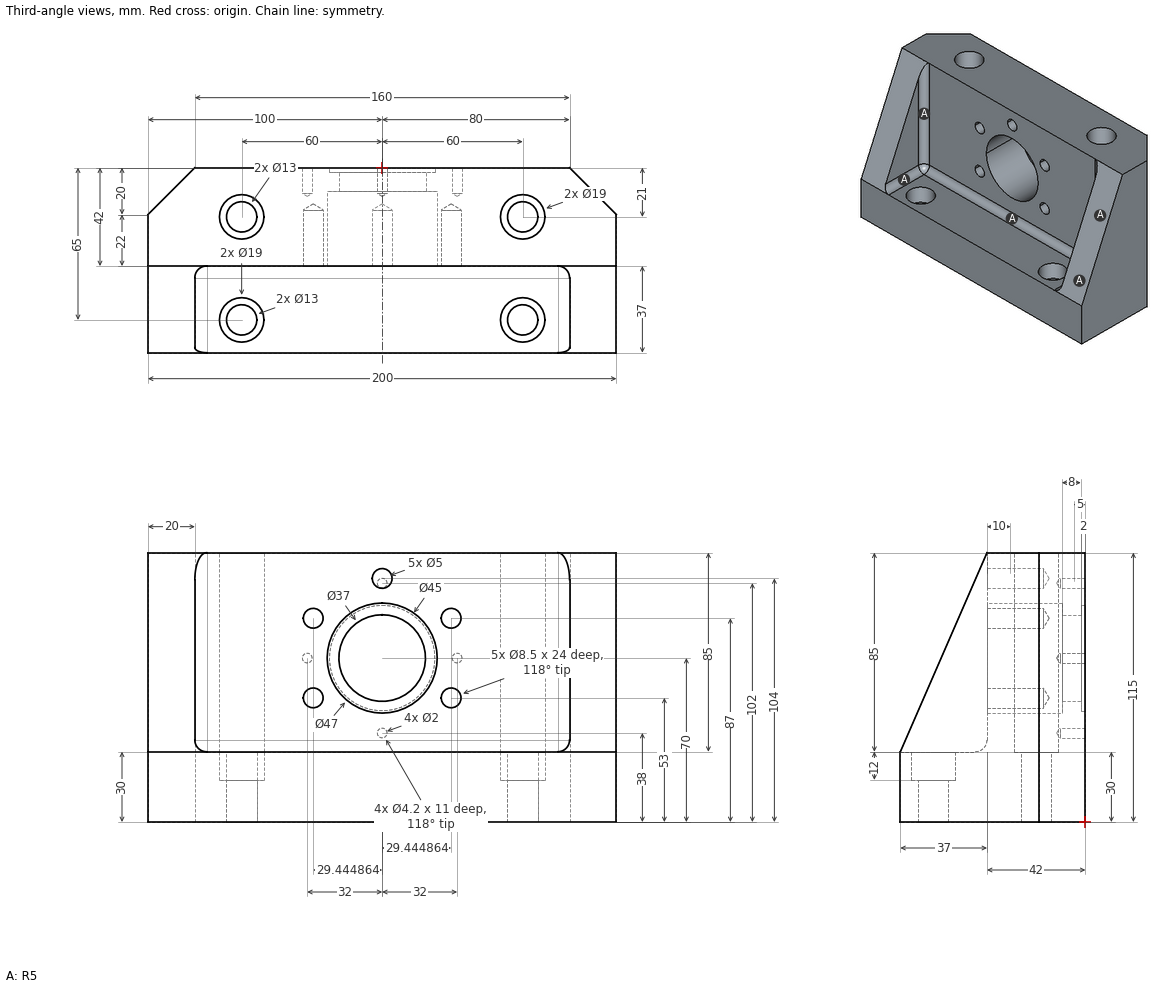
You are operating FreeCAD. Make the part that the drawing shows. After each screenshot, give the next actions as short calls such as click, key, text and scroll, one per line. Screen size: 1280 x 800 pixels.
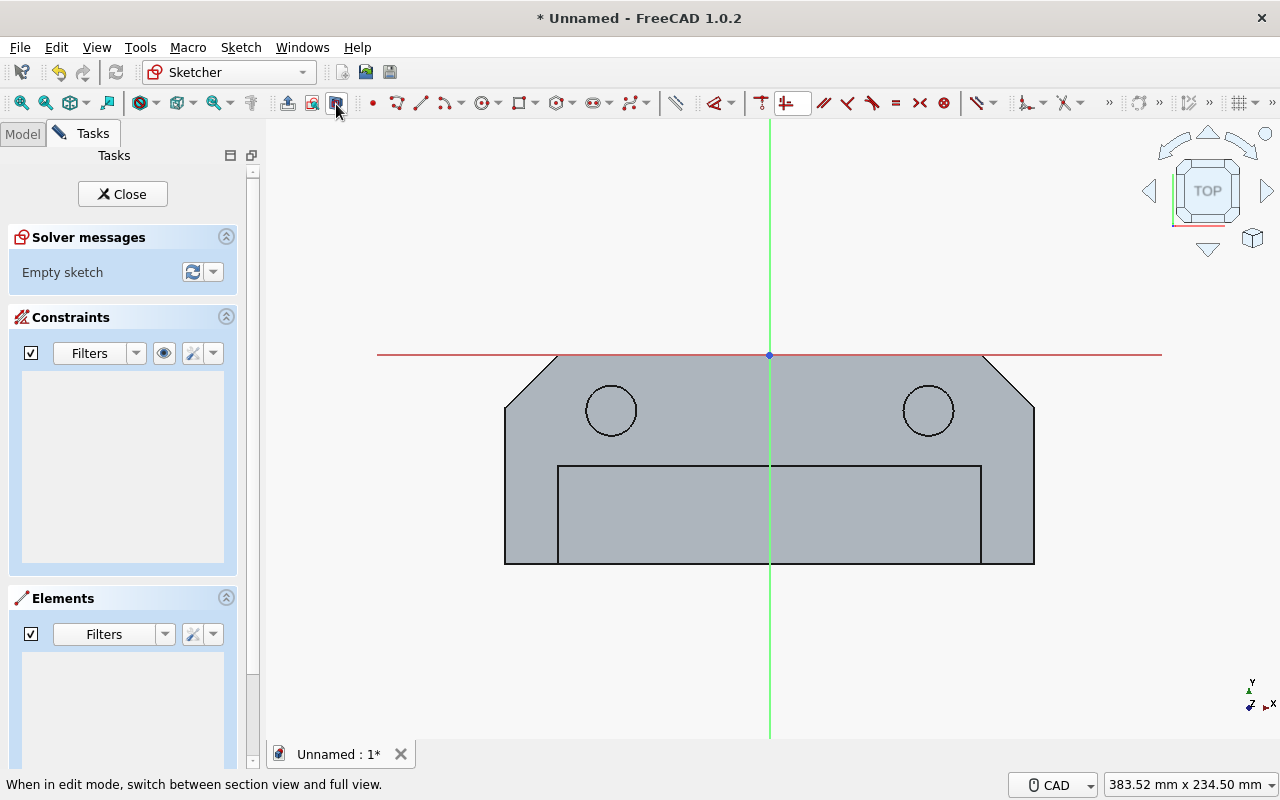
scroll(903, 315, up, 2)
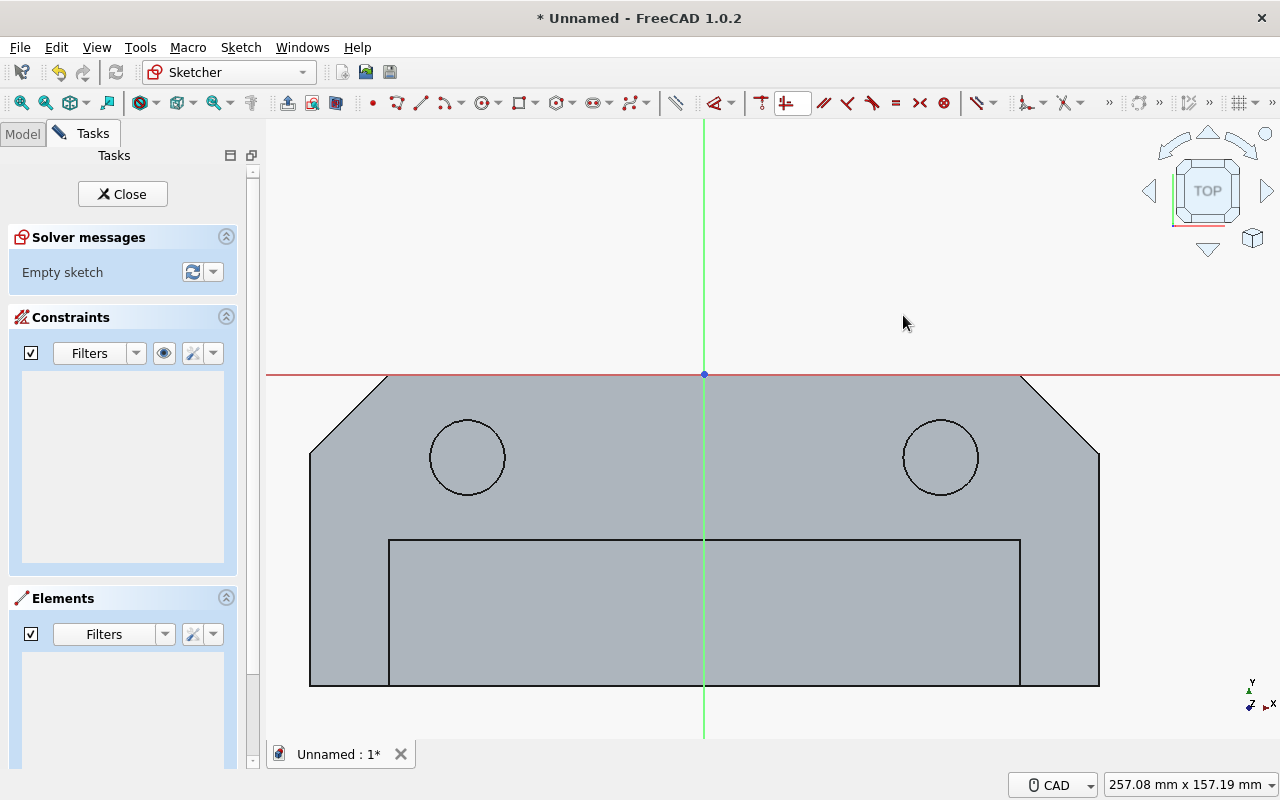
click(482, 104)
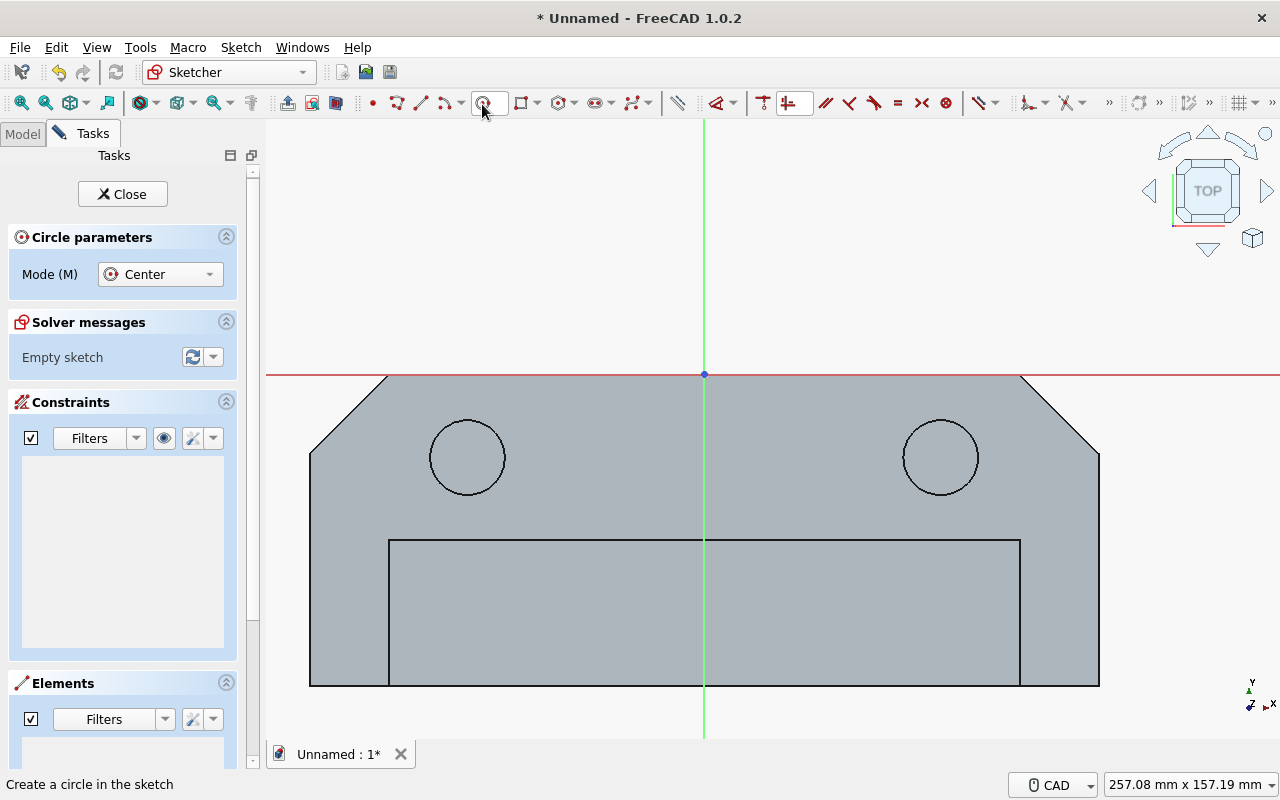
click(467, 458)
move(486, 440)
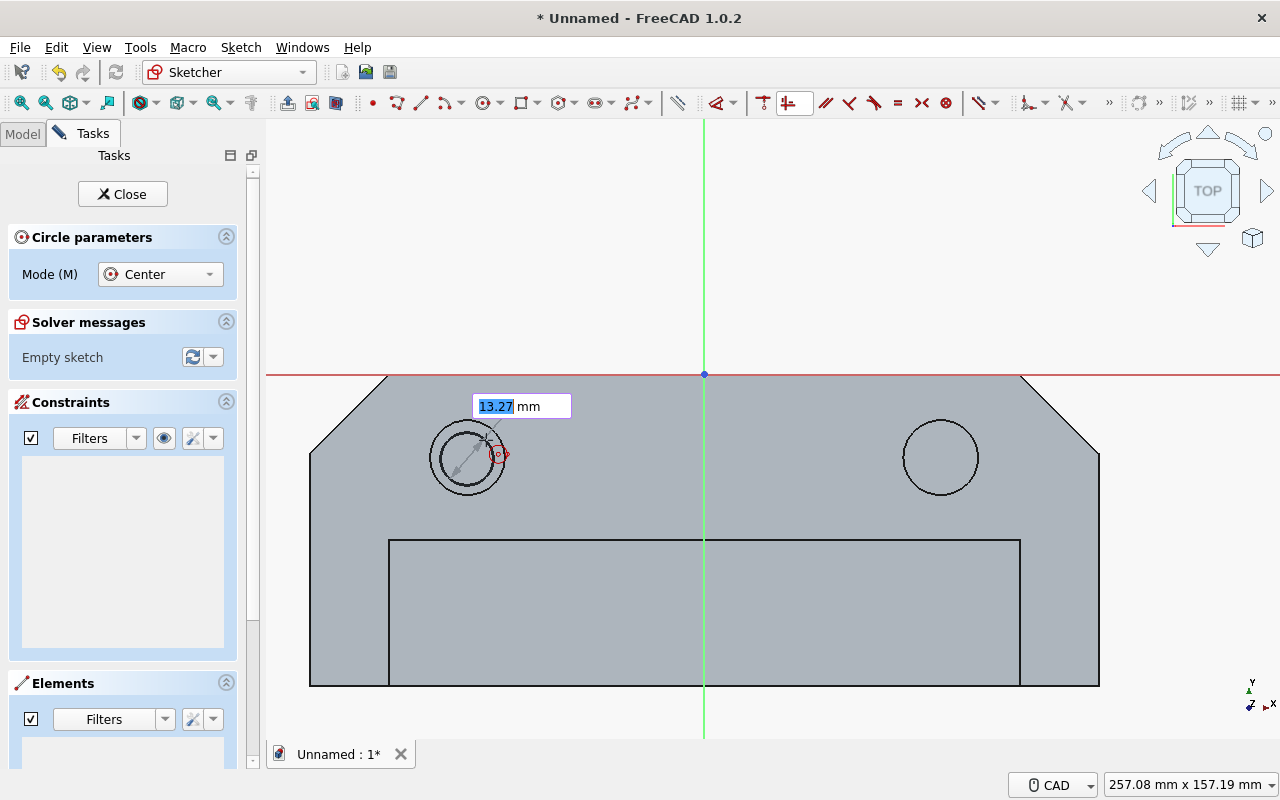
text(13)
key(Return)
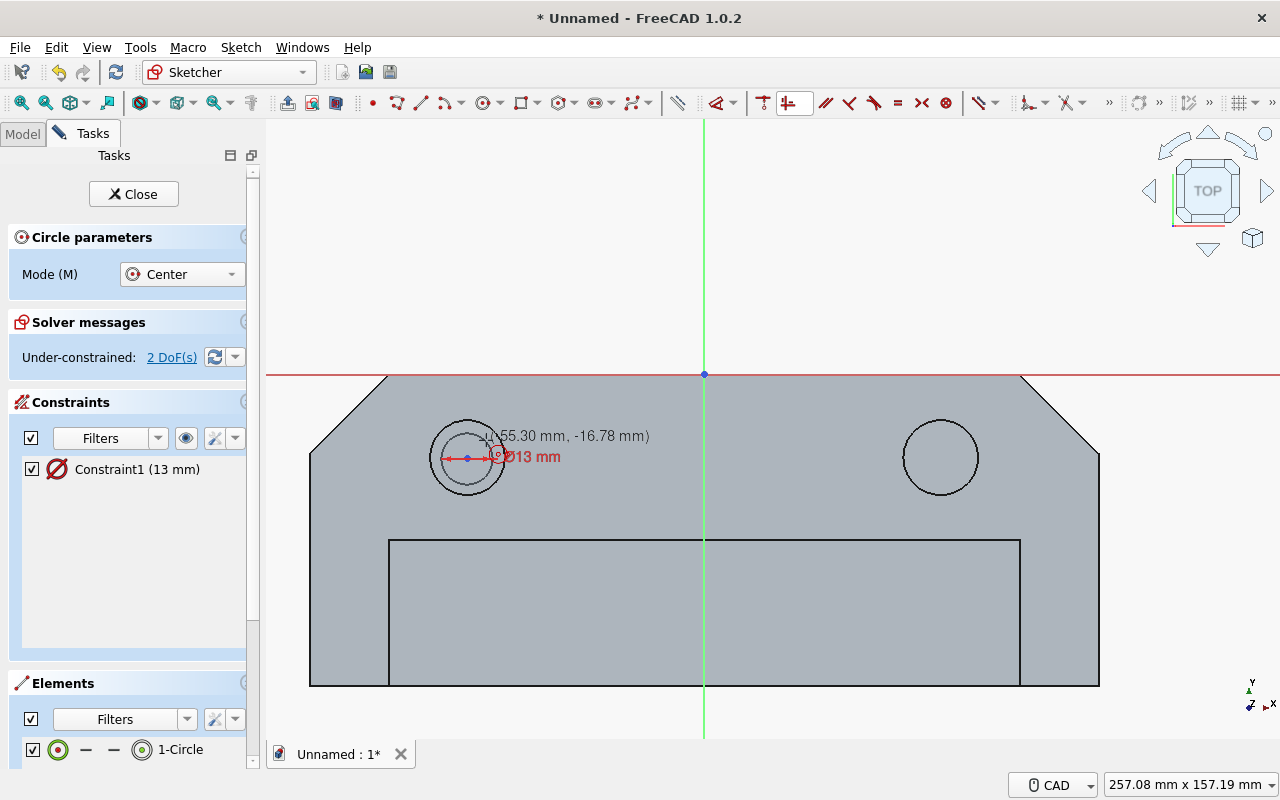
click(941, 458)
move(959, 440)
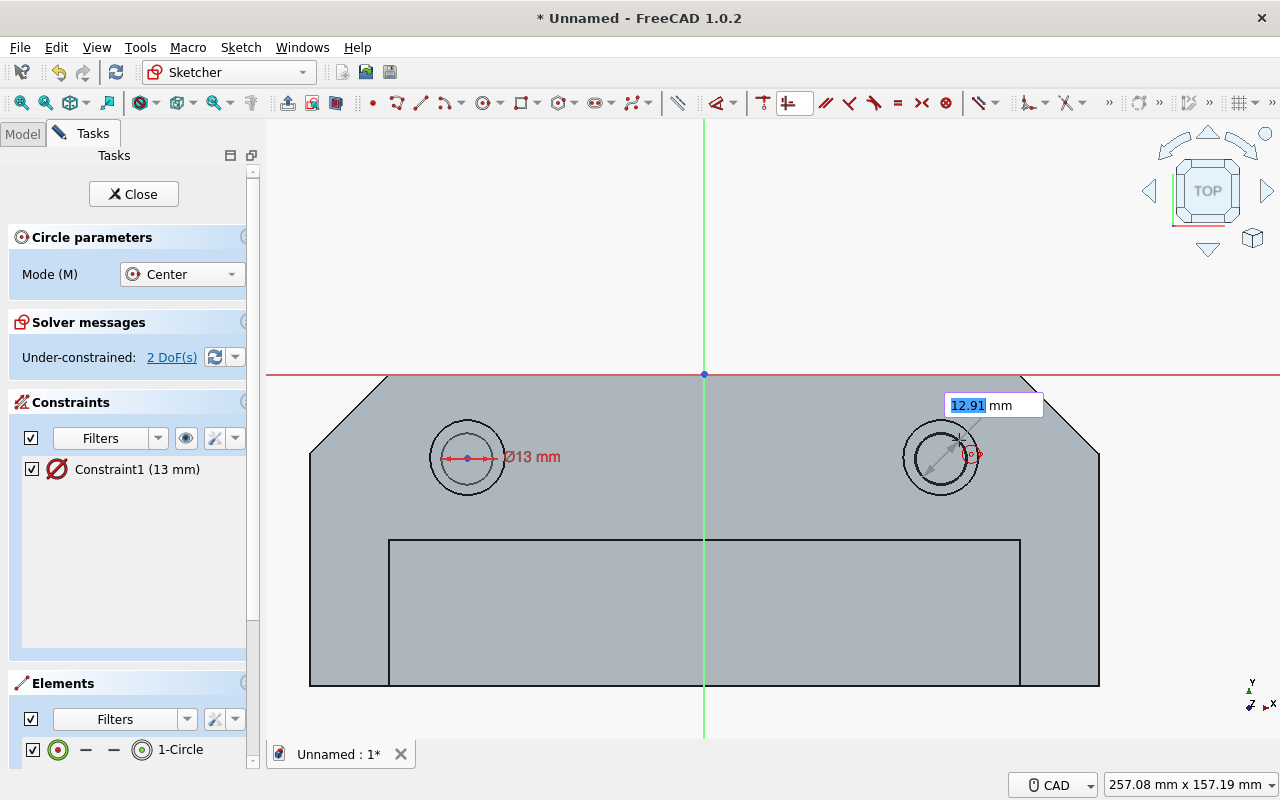
text(13)
key(Return)
key(Escape)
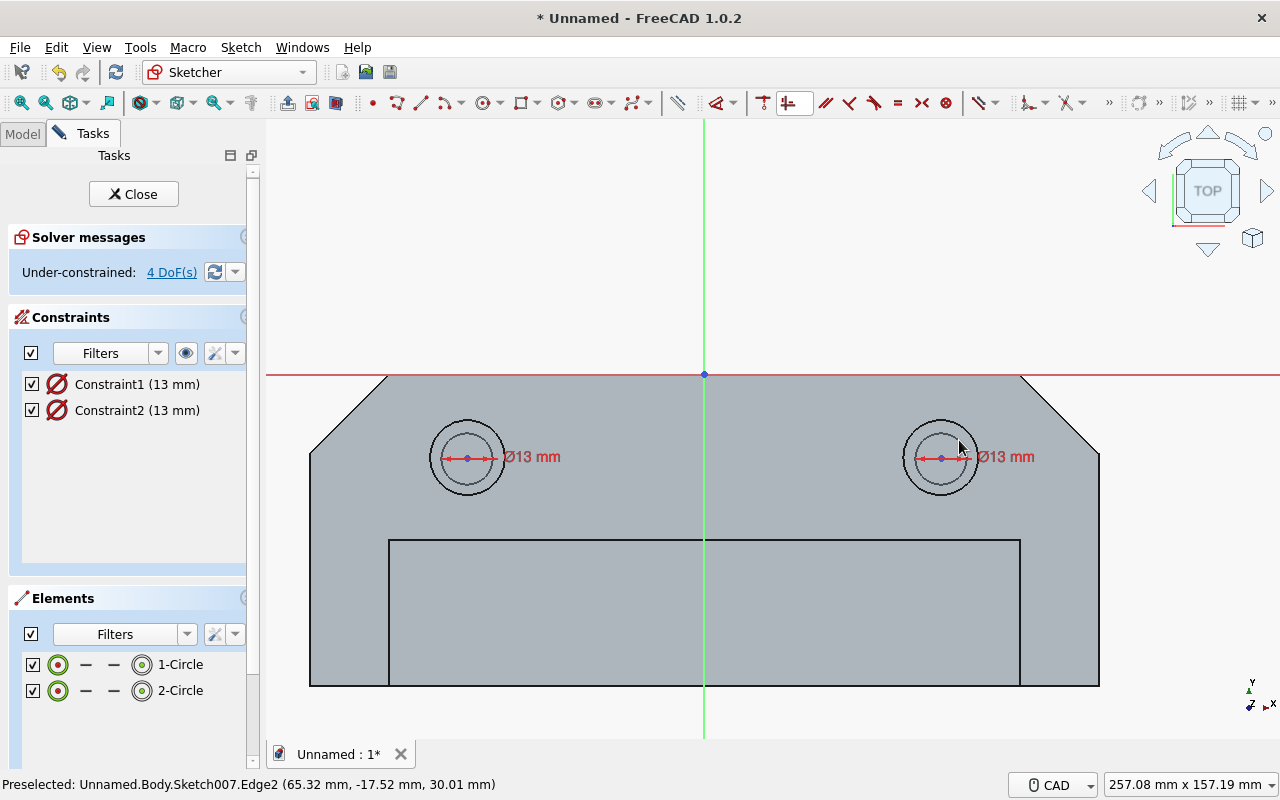
click(467, 459)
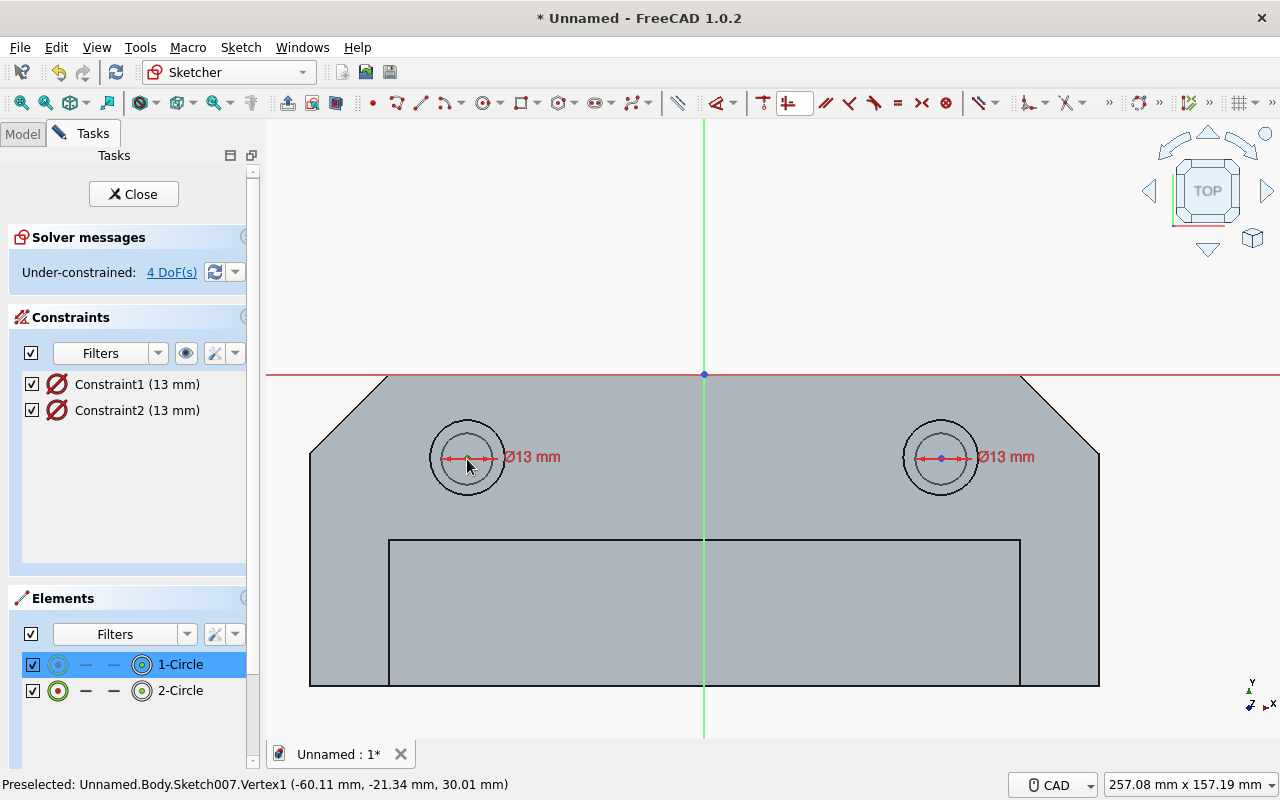
click(941, 459)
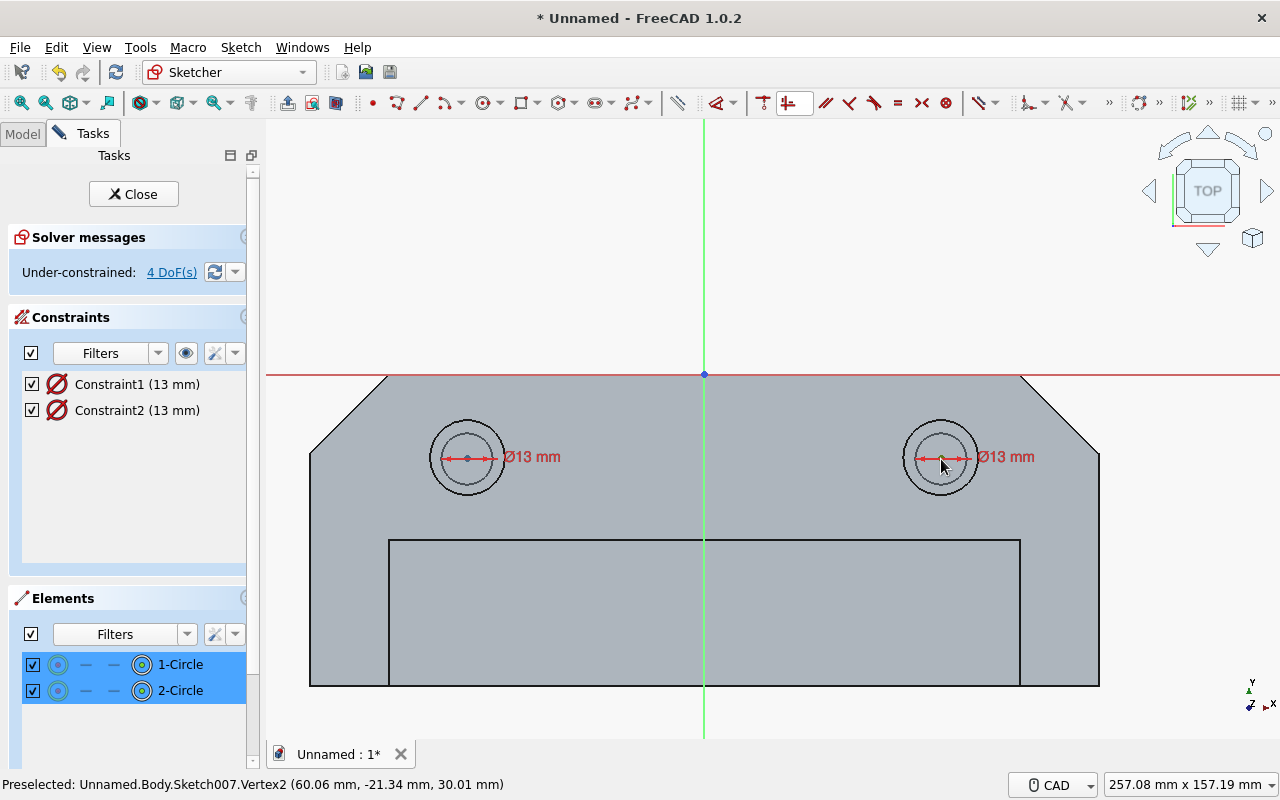
key(h)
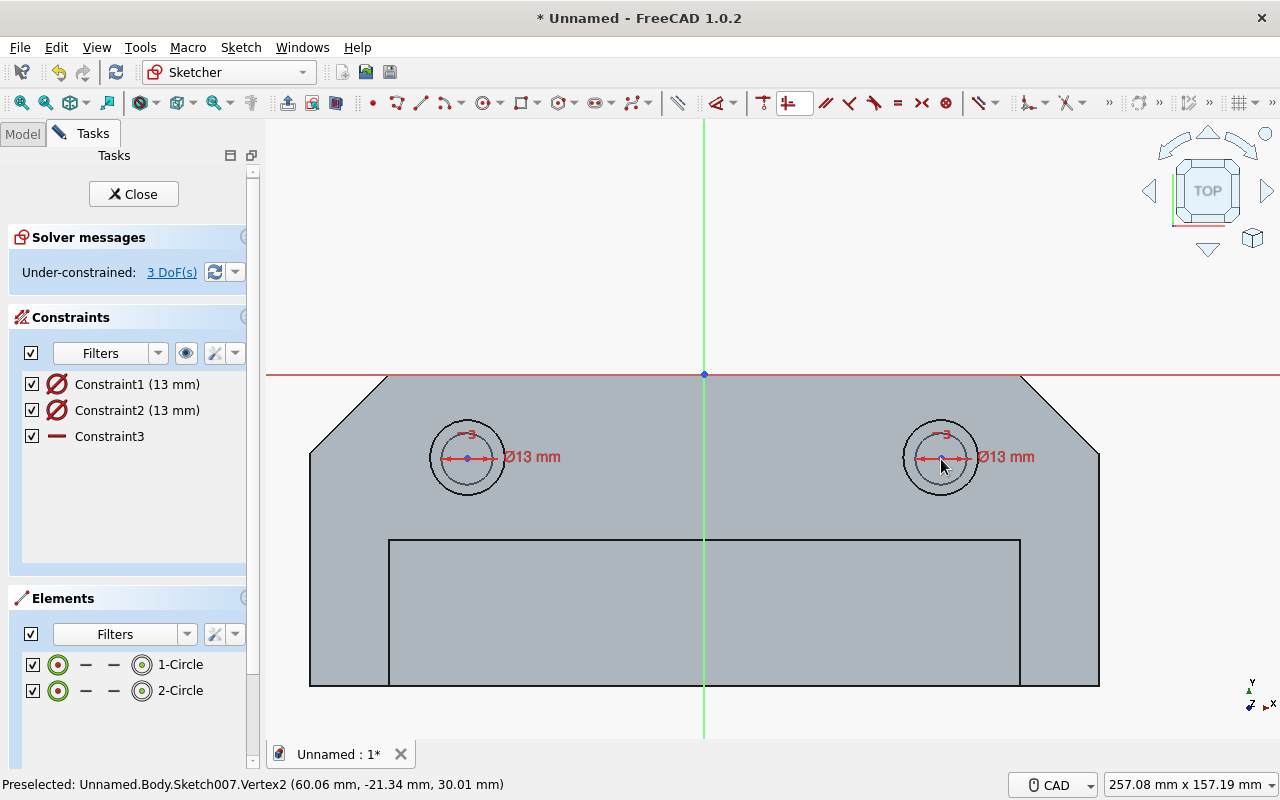
click(716, 104)